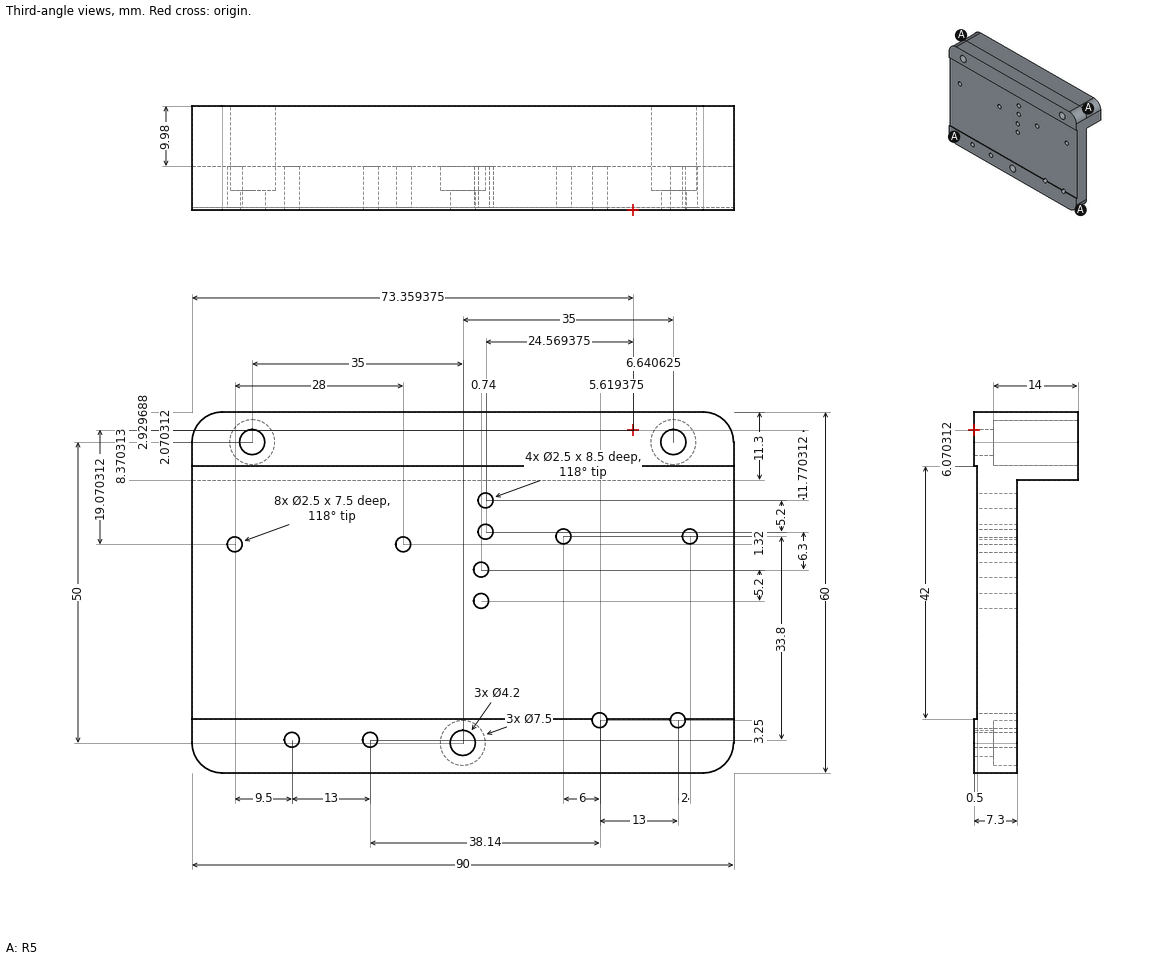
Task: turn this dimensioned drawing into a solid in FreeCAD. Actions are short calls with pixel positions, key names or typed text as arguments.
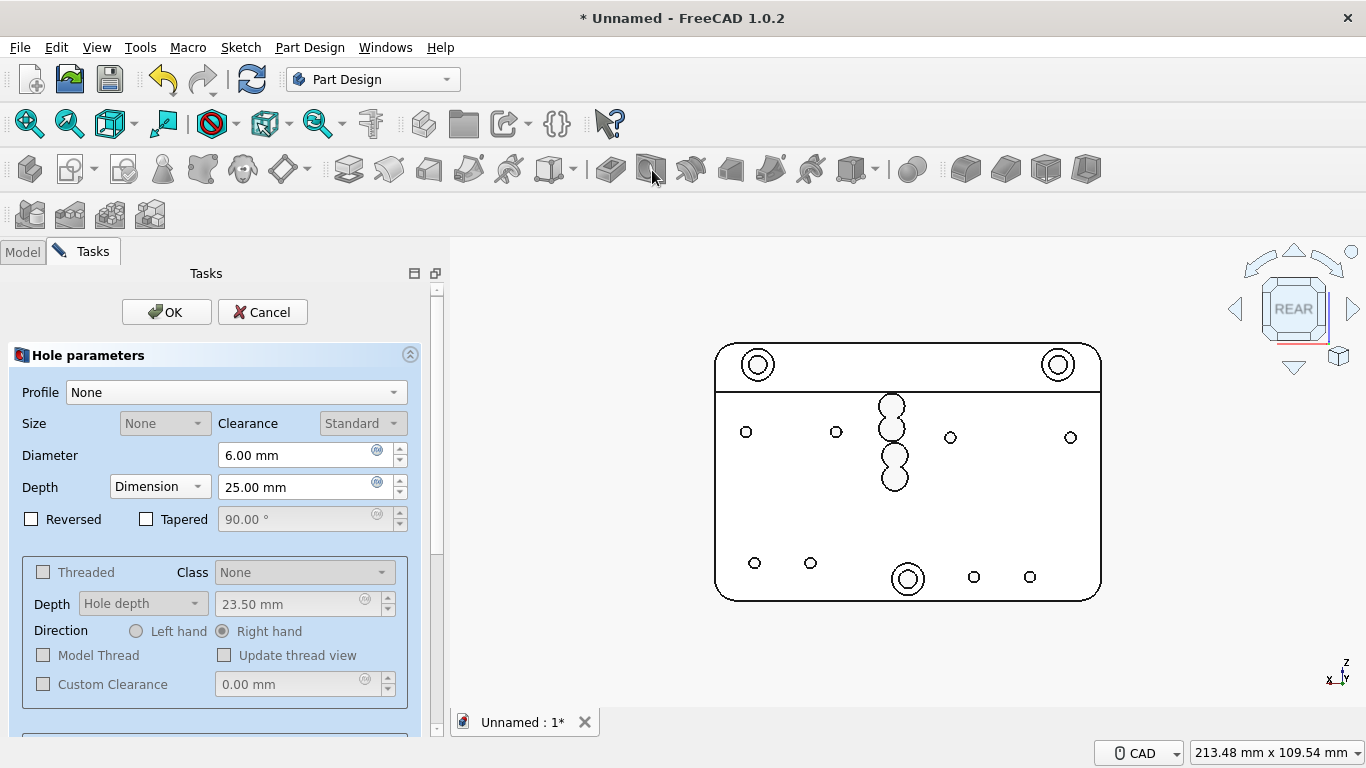
triple_click(305, 455)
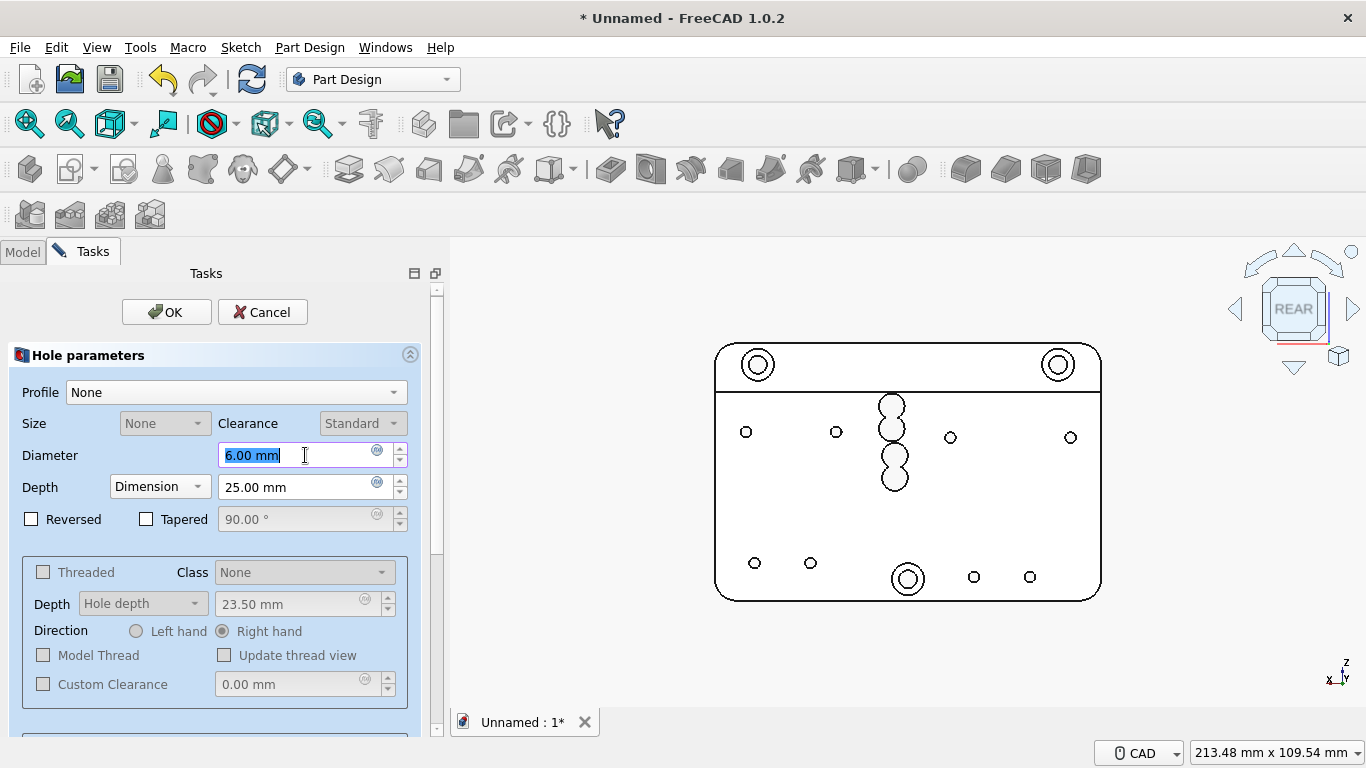
text(2.5)
key(Tab)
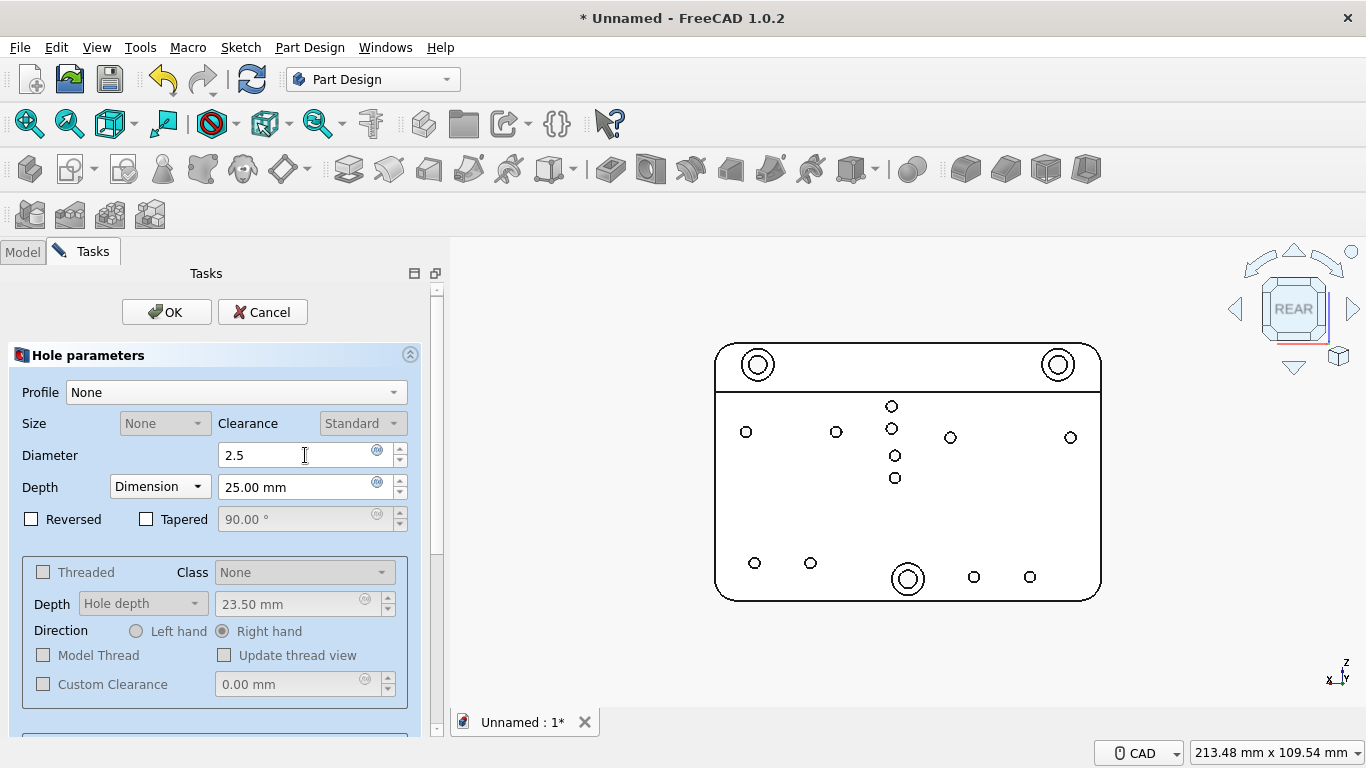
triple_click(305, 487)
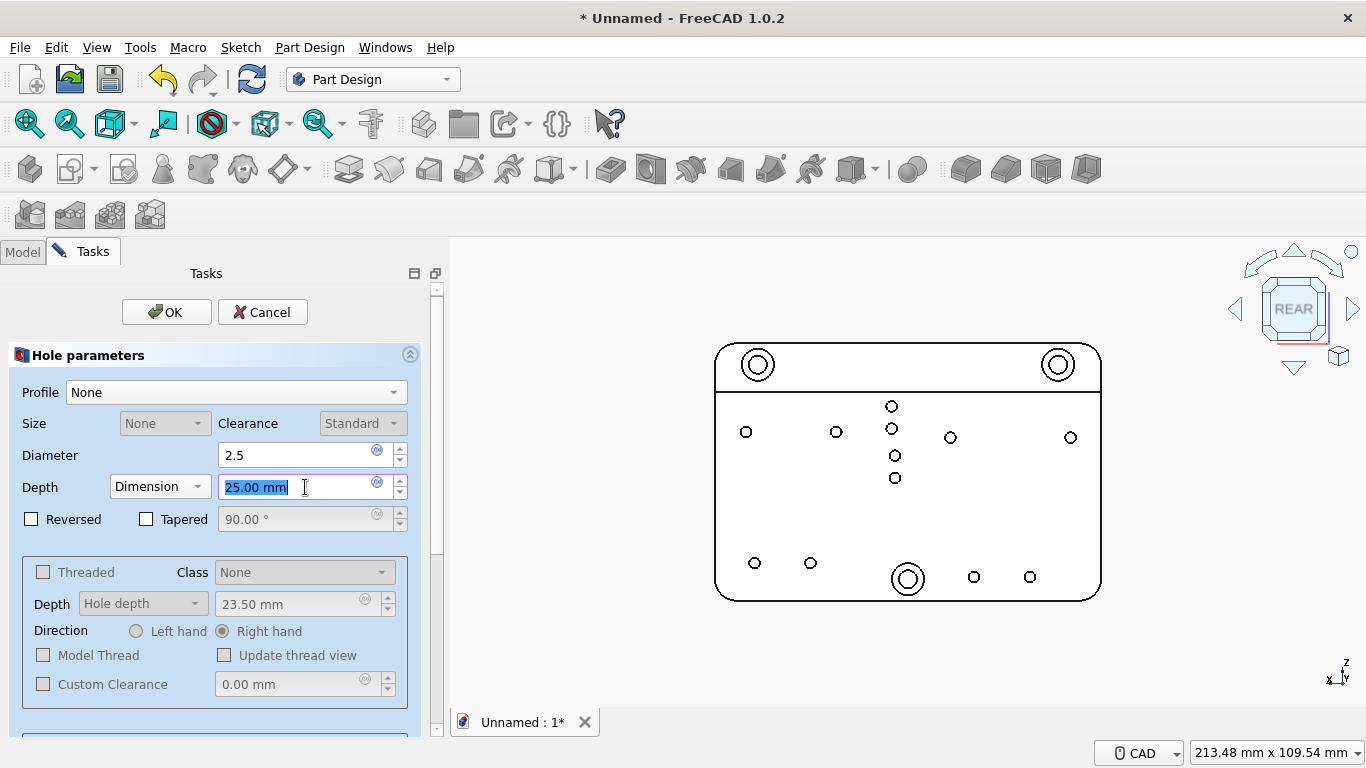
text(8.5)
key(Tab)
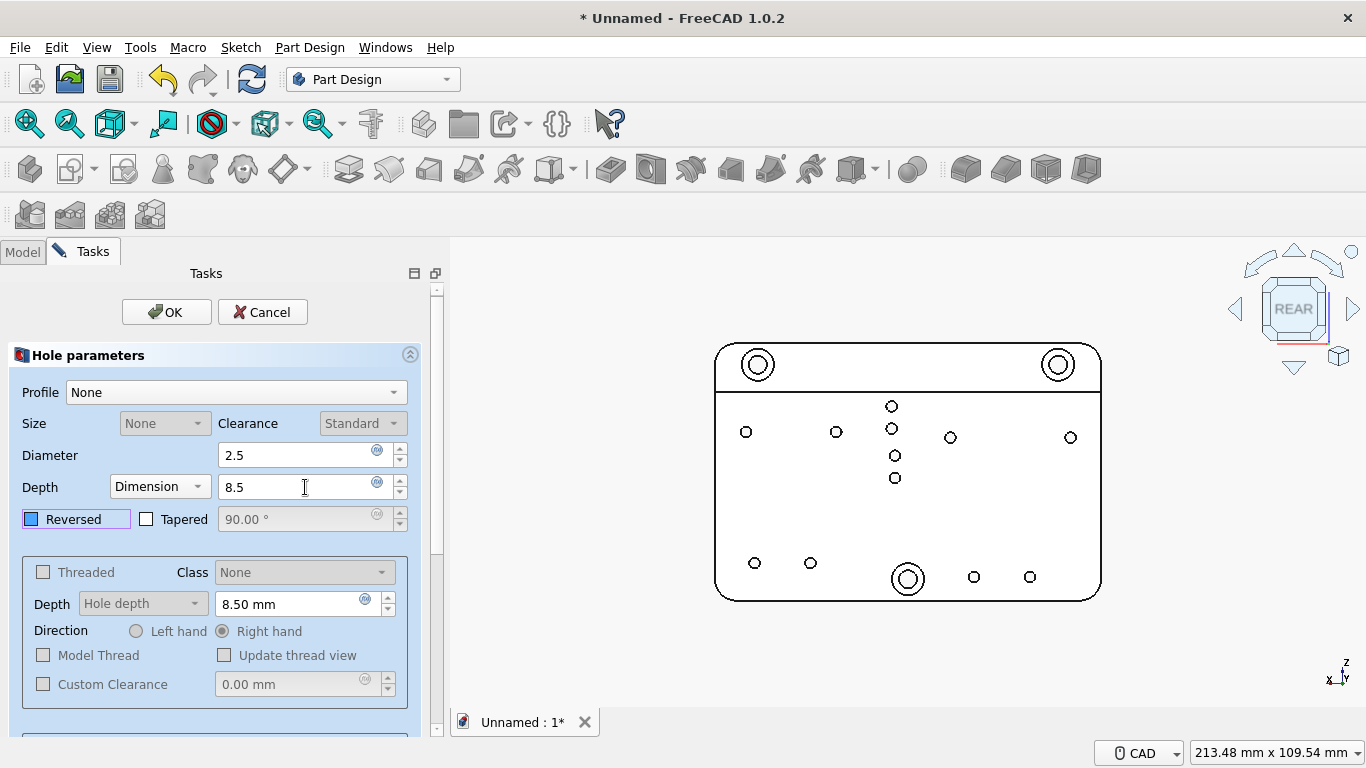
click(167, 312)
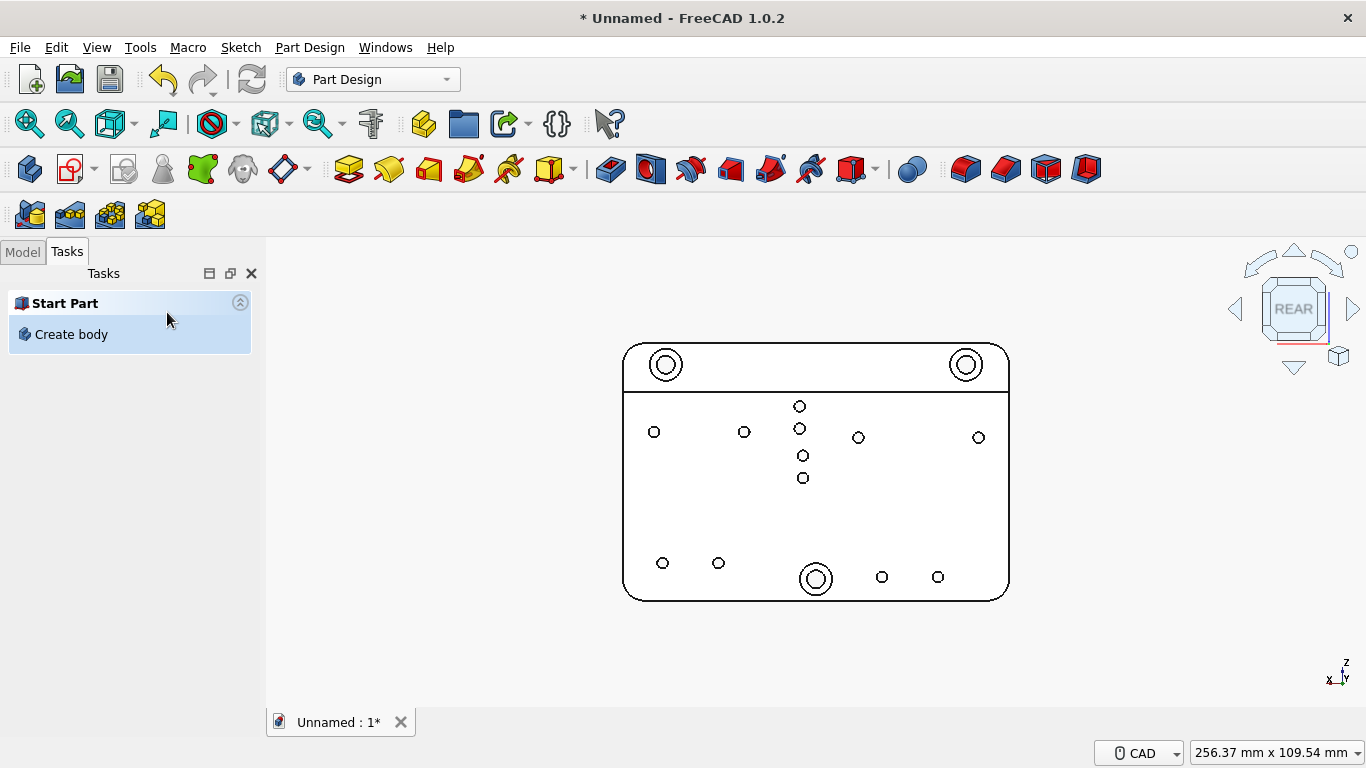
key(0)